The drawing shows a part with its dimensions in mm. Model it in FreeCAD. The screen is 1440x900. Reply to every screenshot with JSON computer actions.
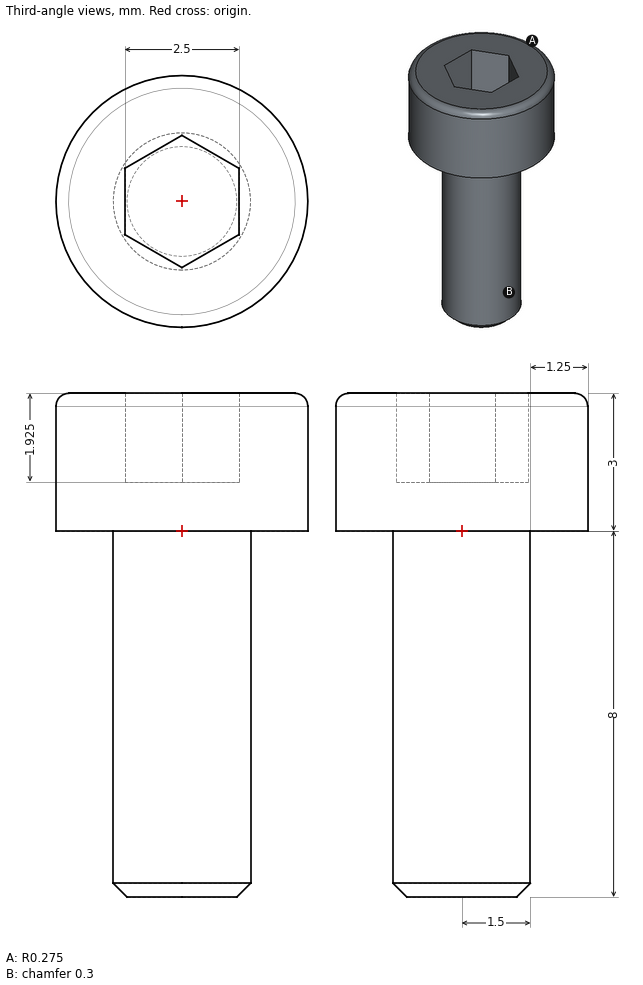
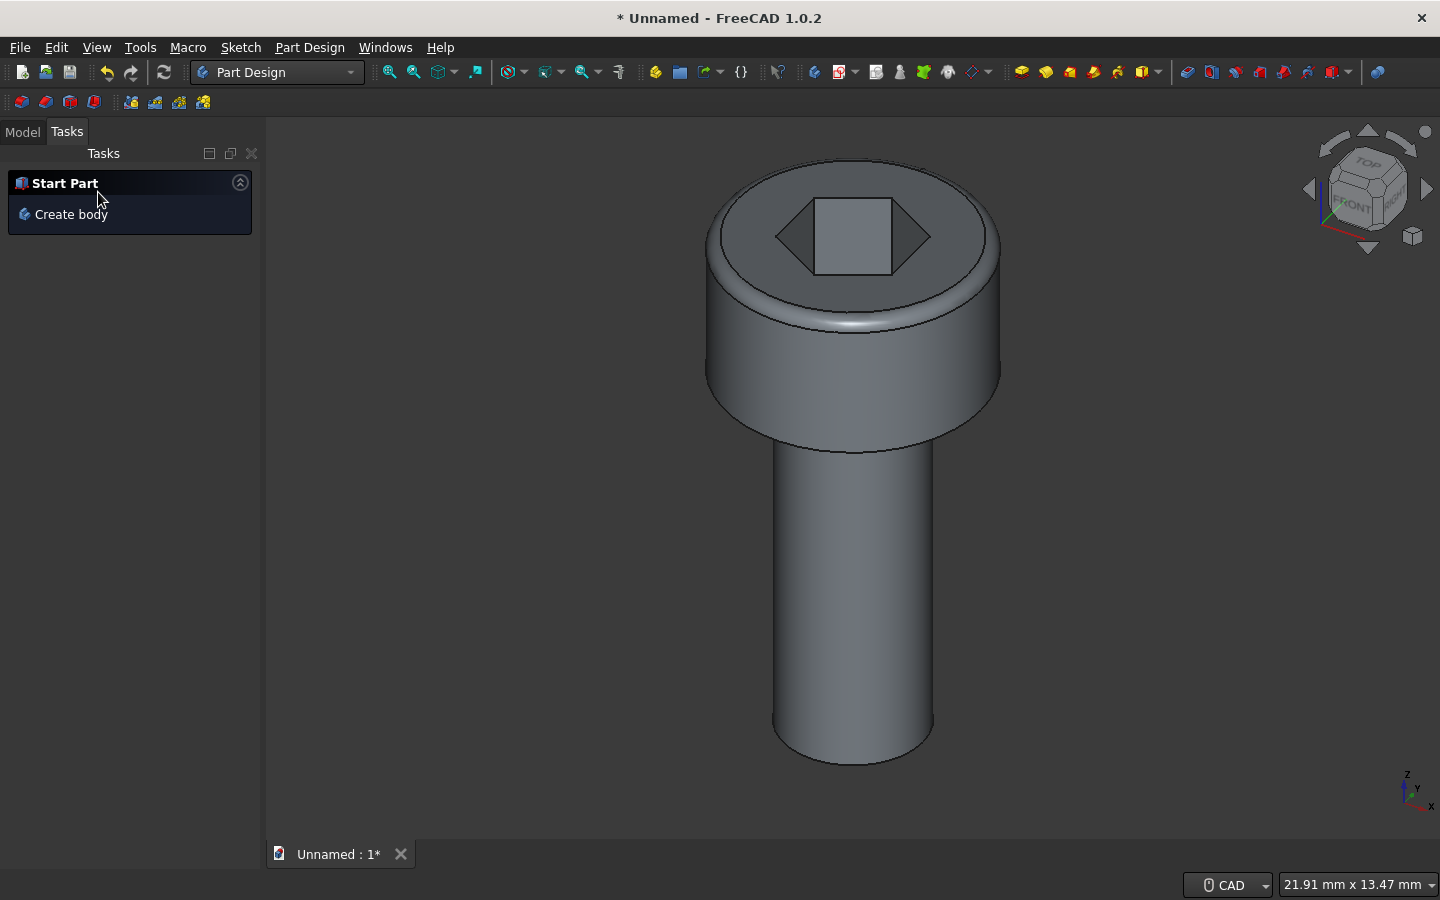
{"action": "key", "text": "0"}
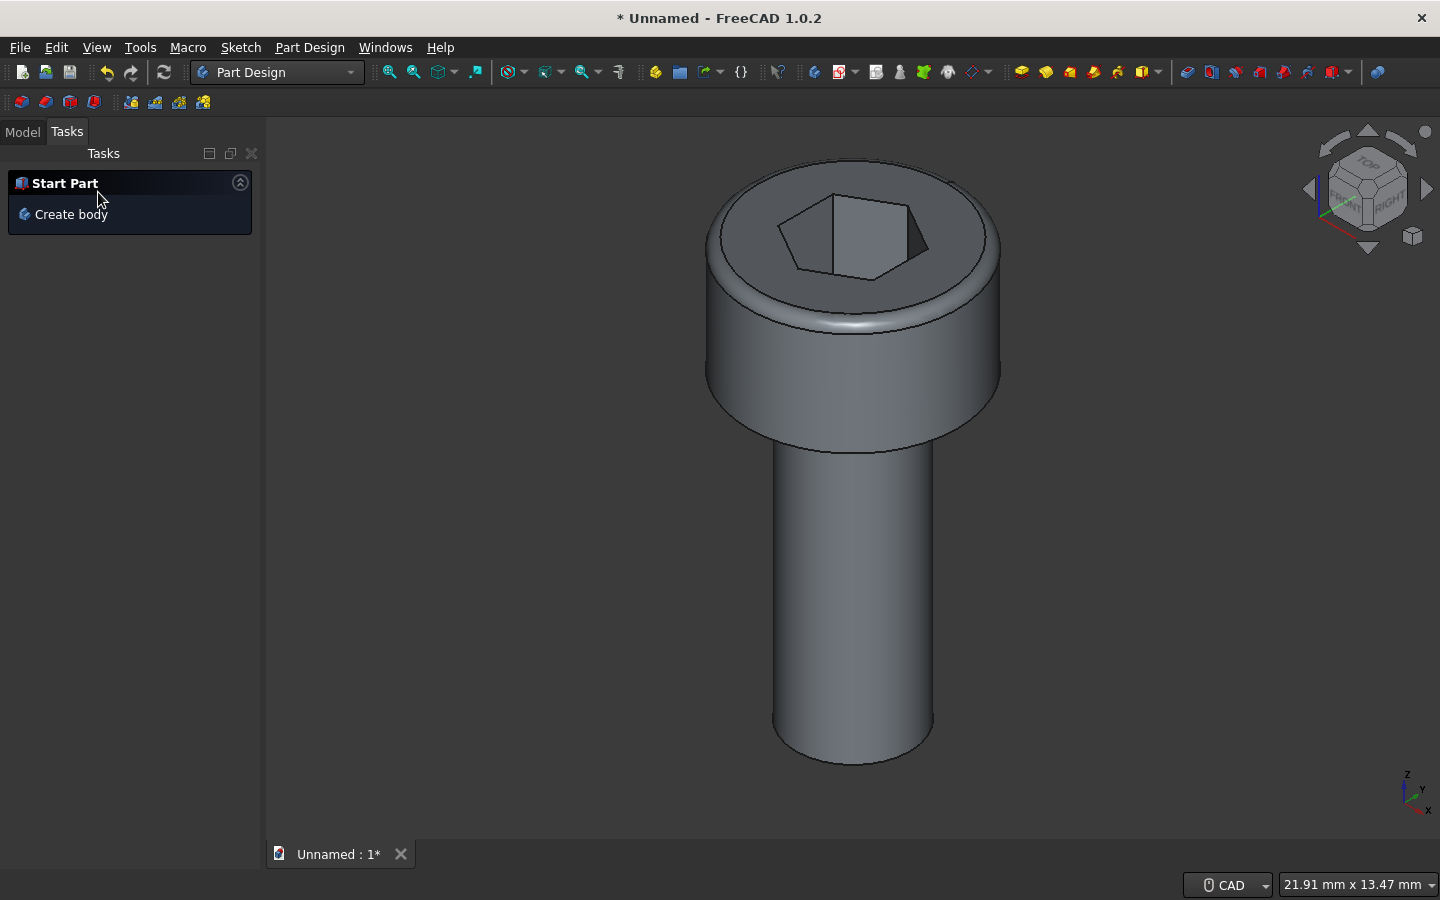
{"action": "left_click", "coordinate": [390, 72]}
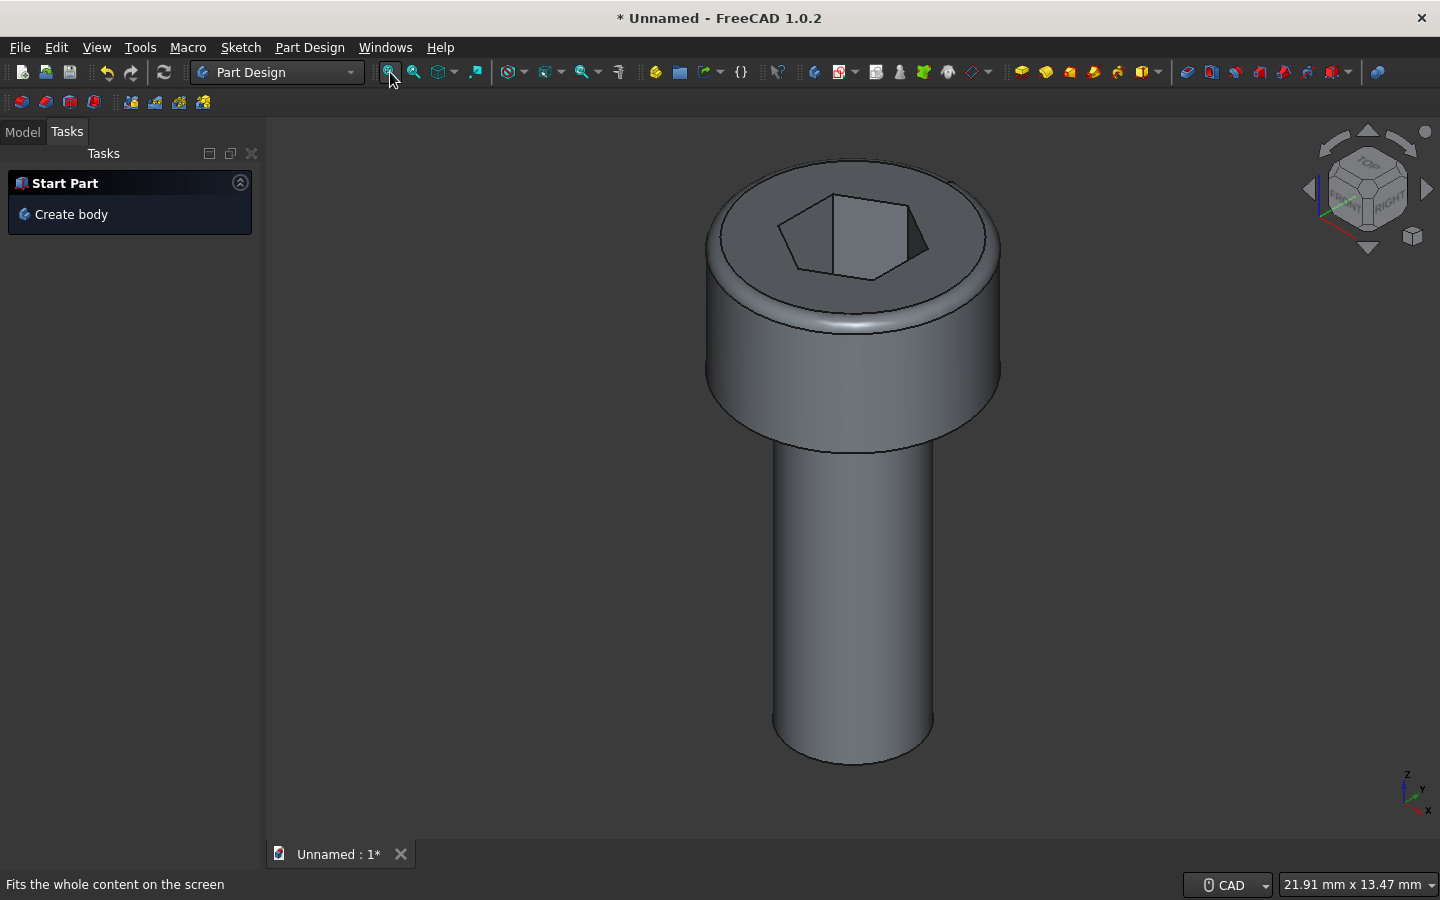
{"action": "key", "text": "2"}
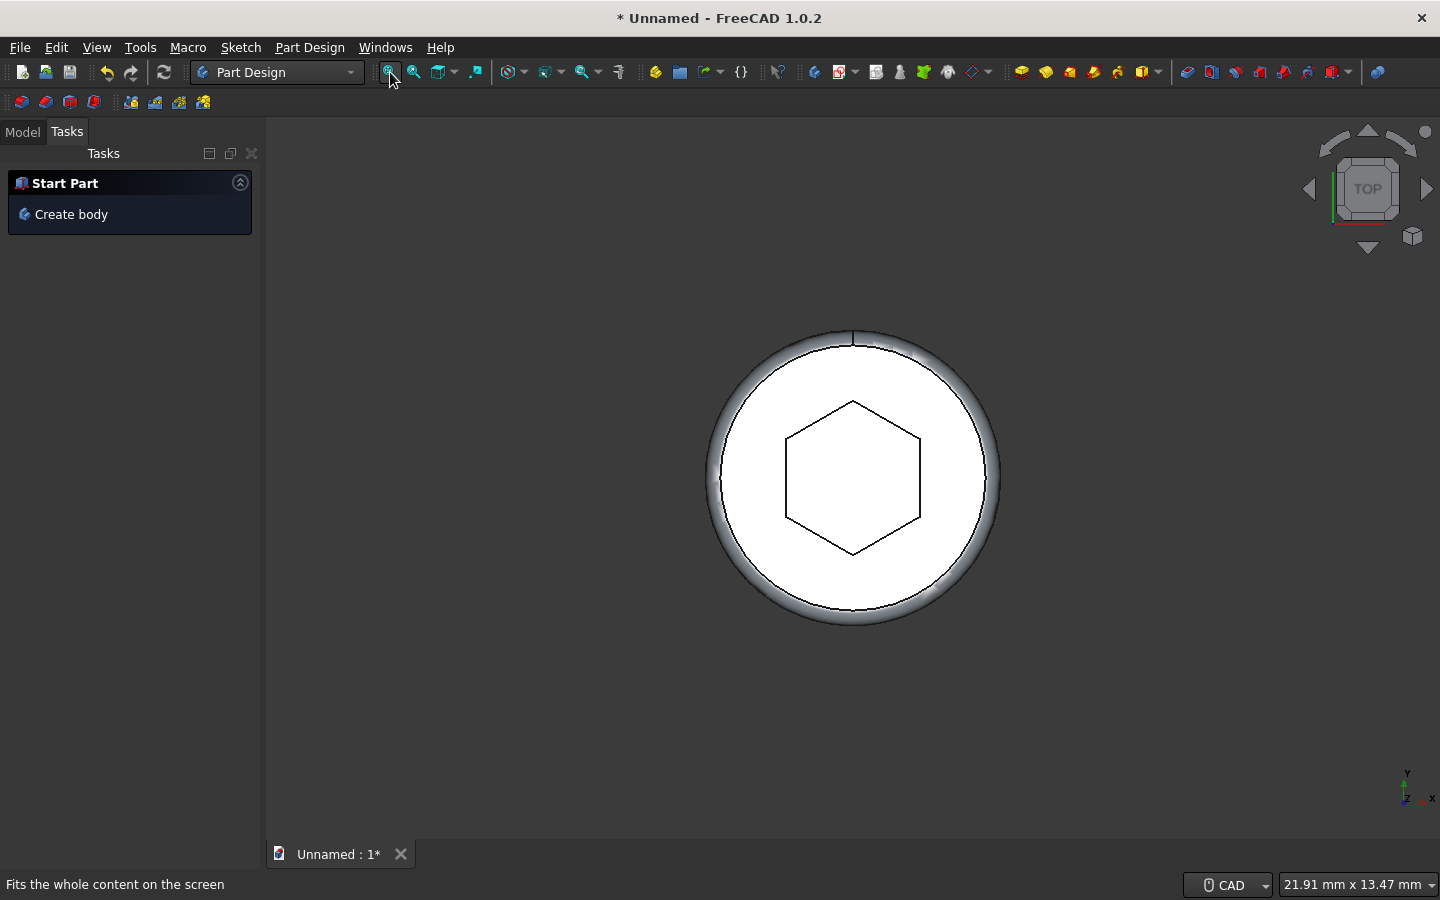
{"action": "left_click", "coordinate": [390, 72]}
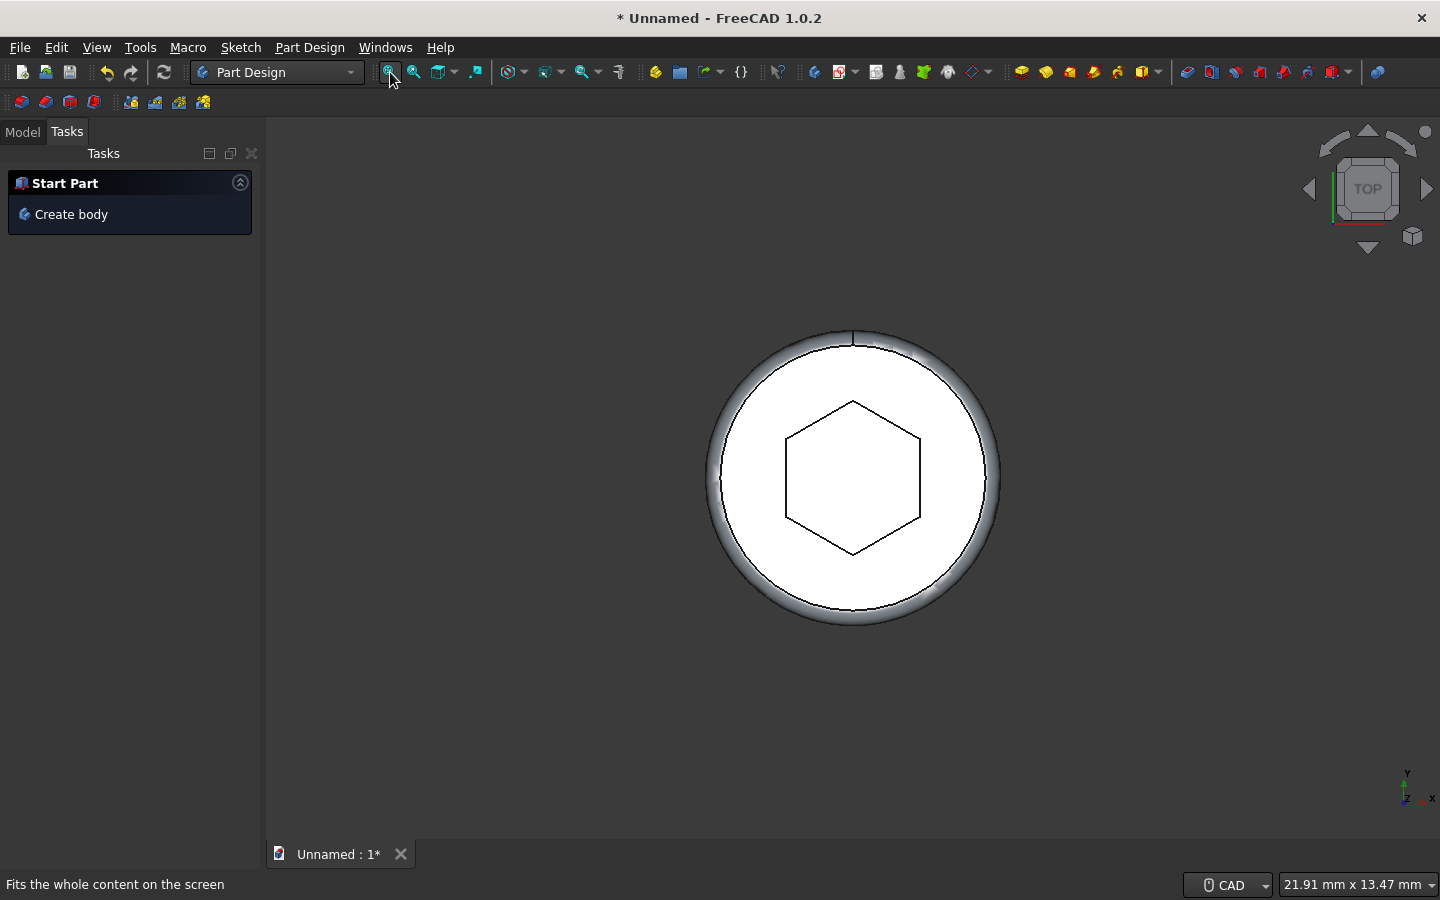
{"action": "key", "text": "1"}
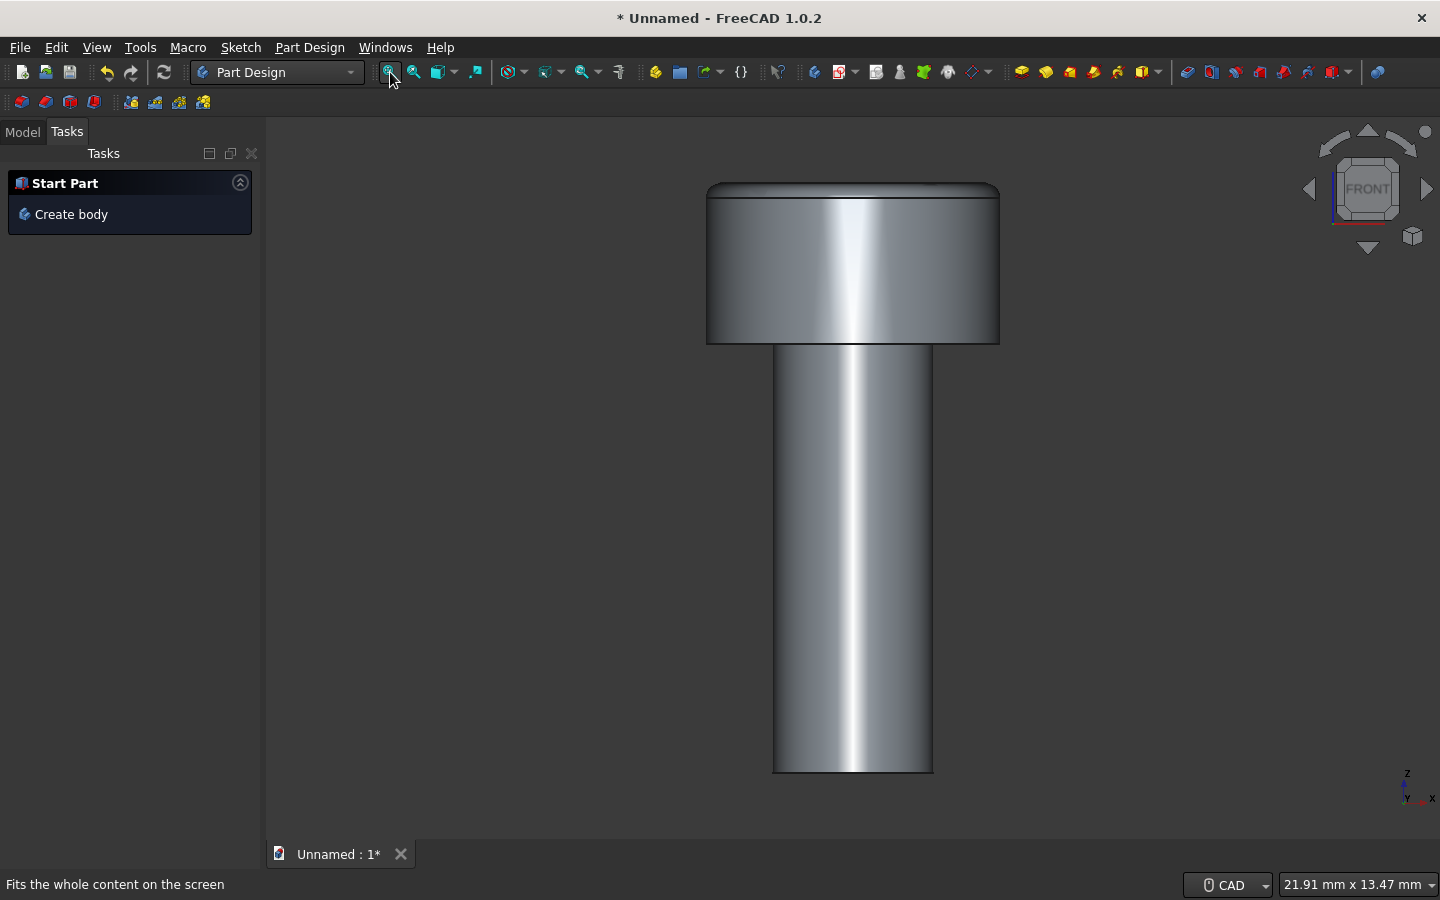
{"action": "left_click", "coordinate": [853, 772]}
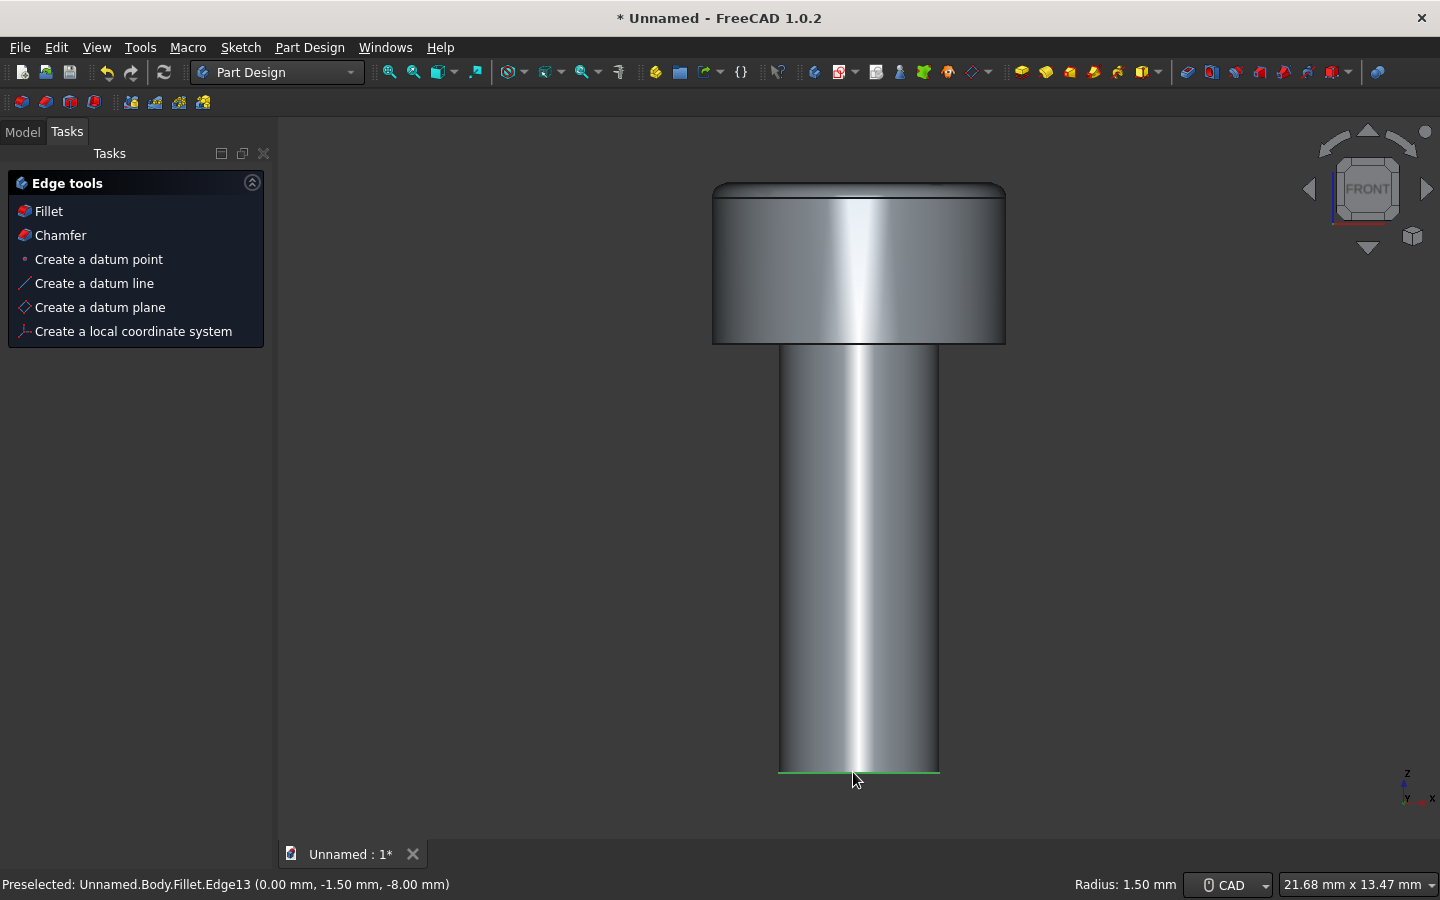
{"action": "left_click", "coordinate": [46, 102]}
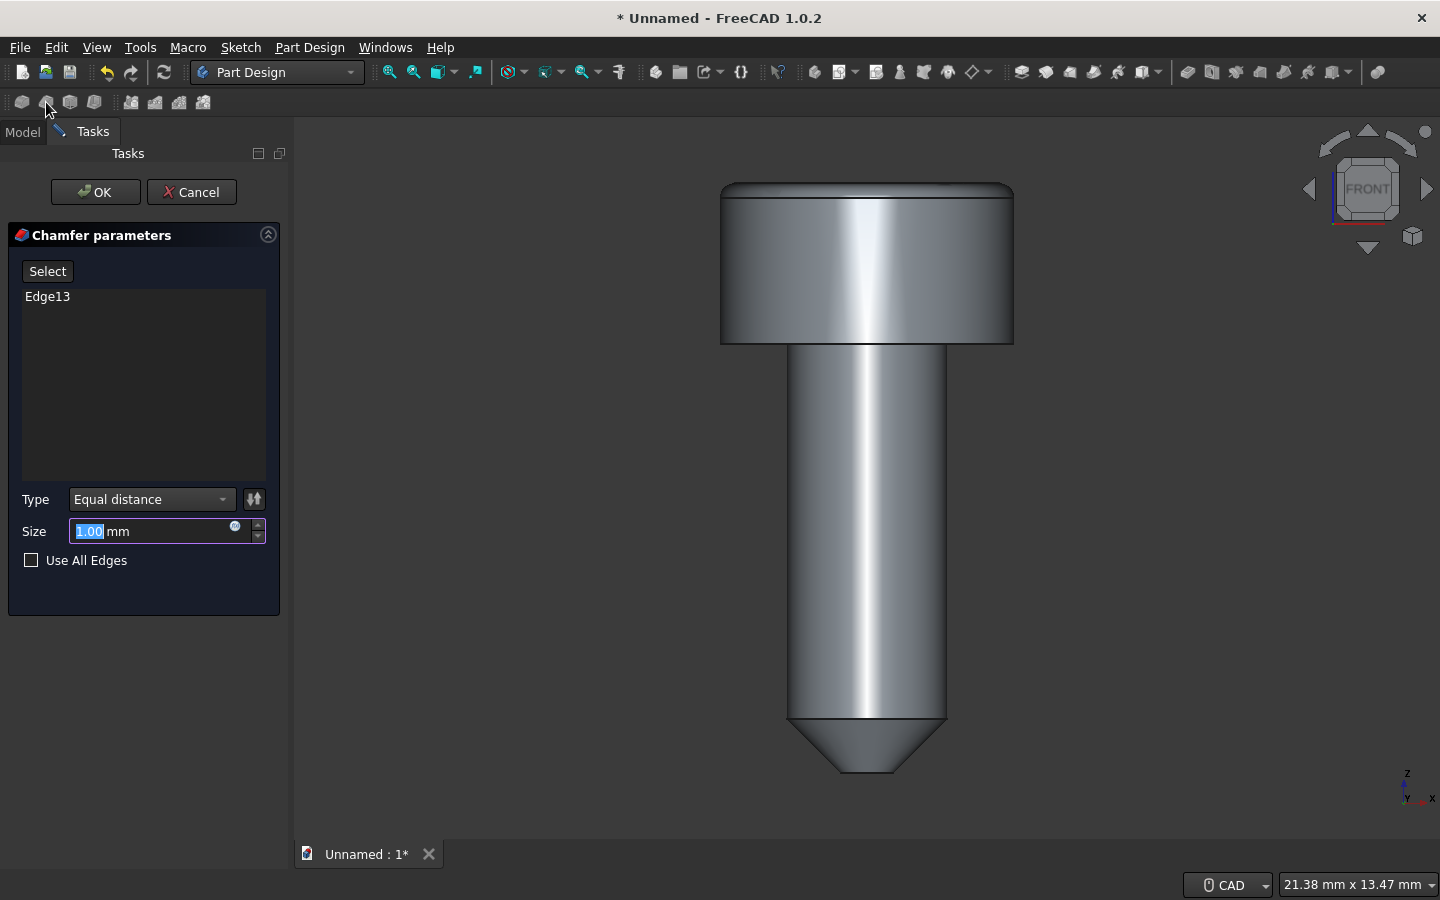
{"action": "type", "text": "0.3"}
{"action": "key", "text": "Tab"}